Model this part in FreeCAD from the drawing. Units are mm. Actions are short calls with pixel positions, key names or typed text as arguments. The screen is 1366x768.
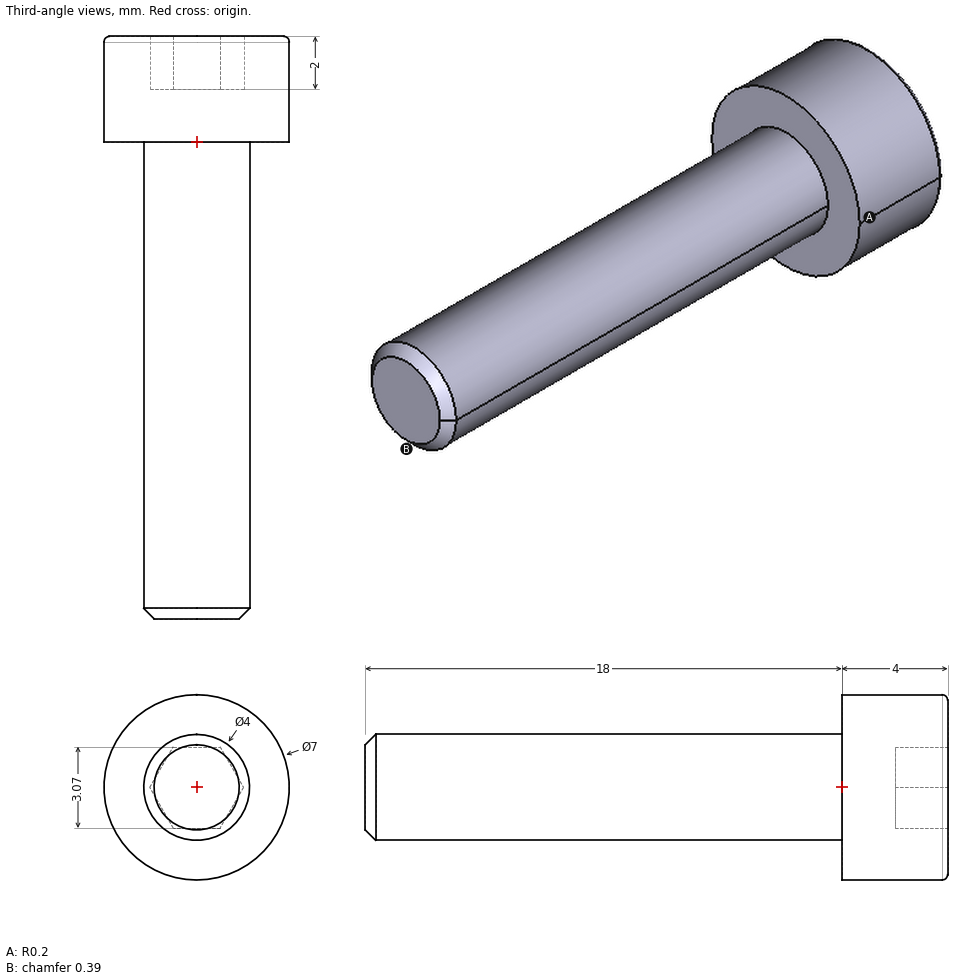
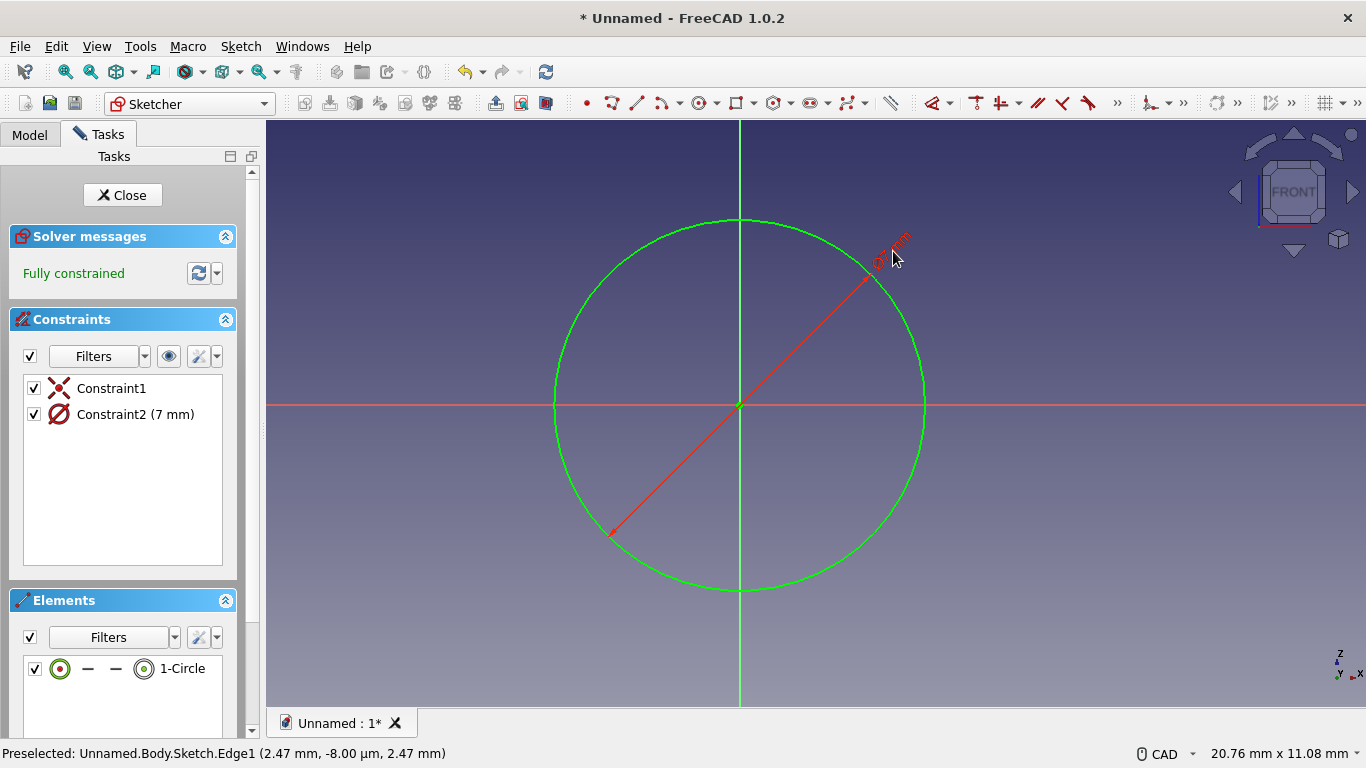
click(123, 195)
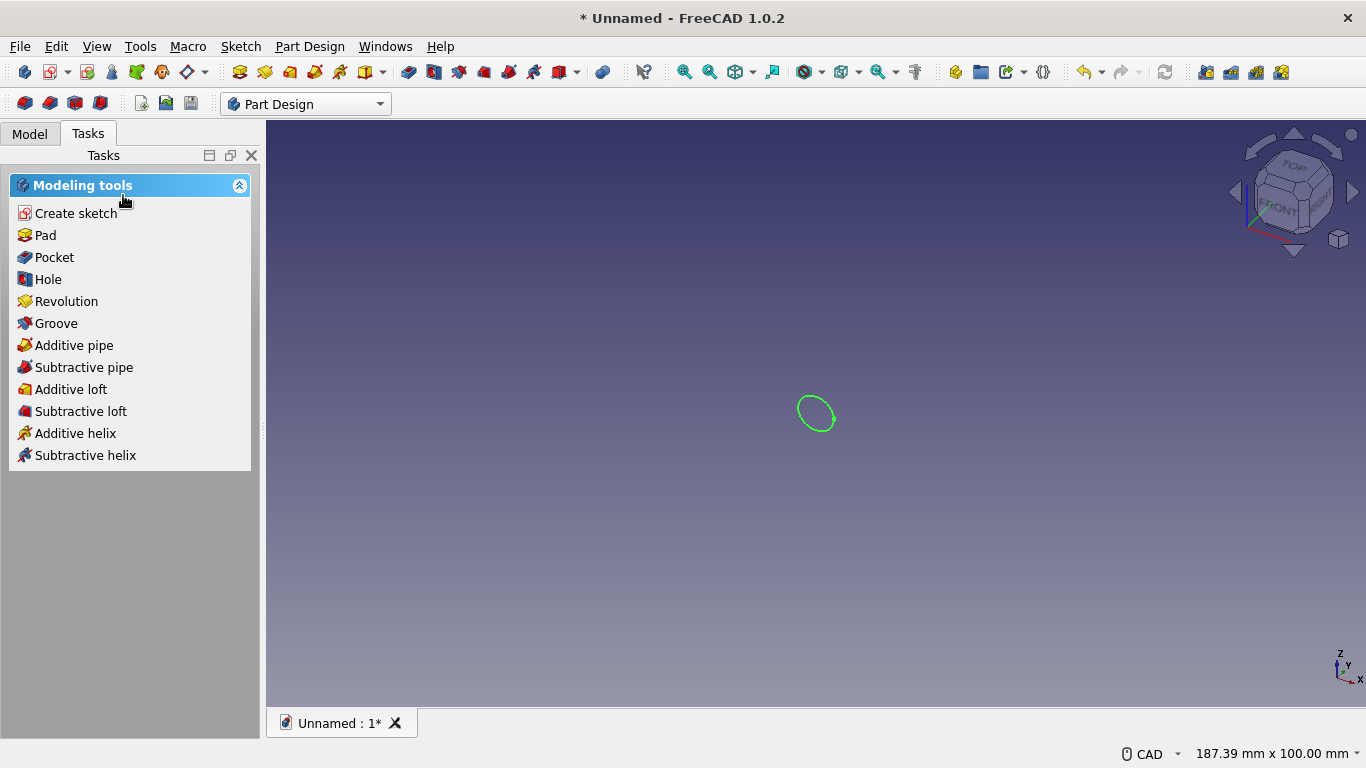
click(240, 72)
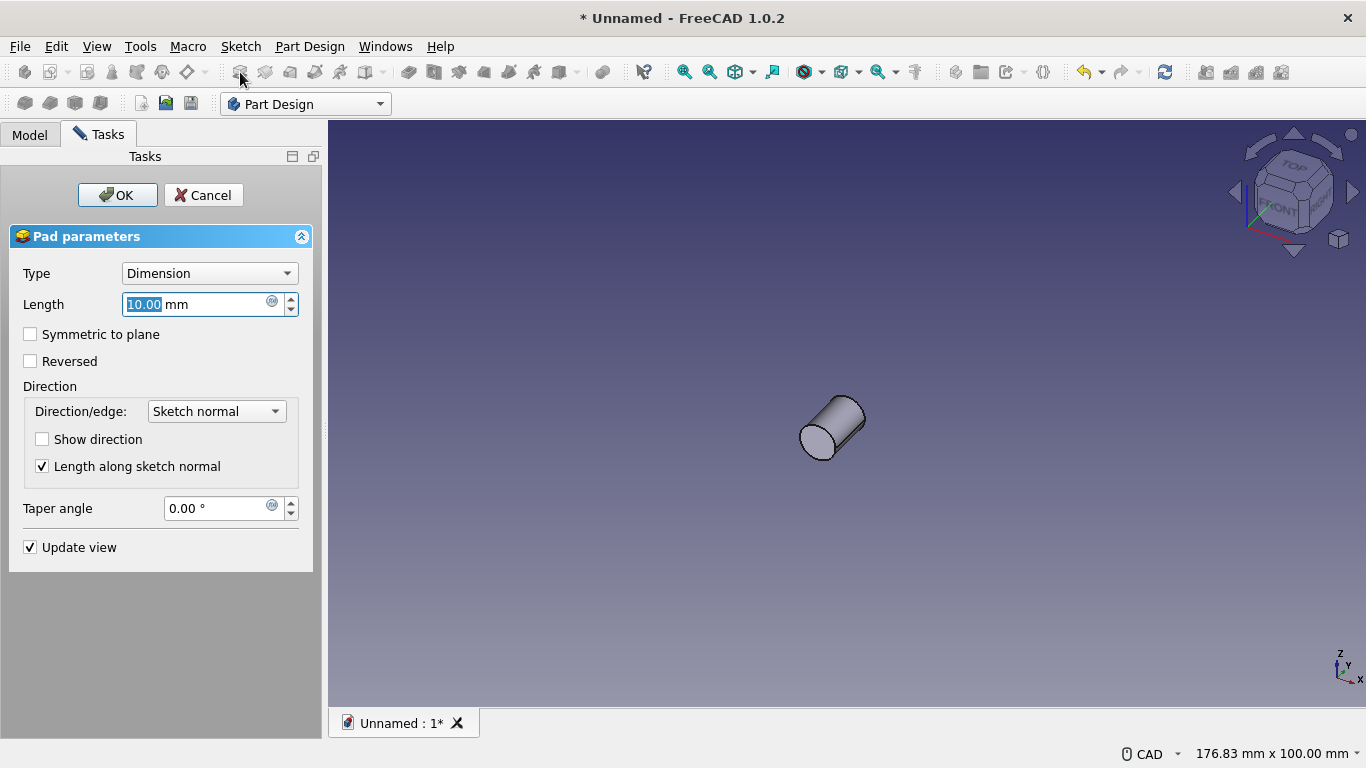
text(4)
key(Tab)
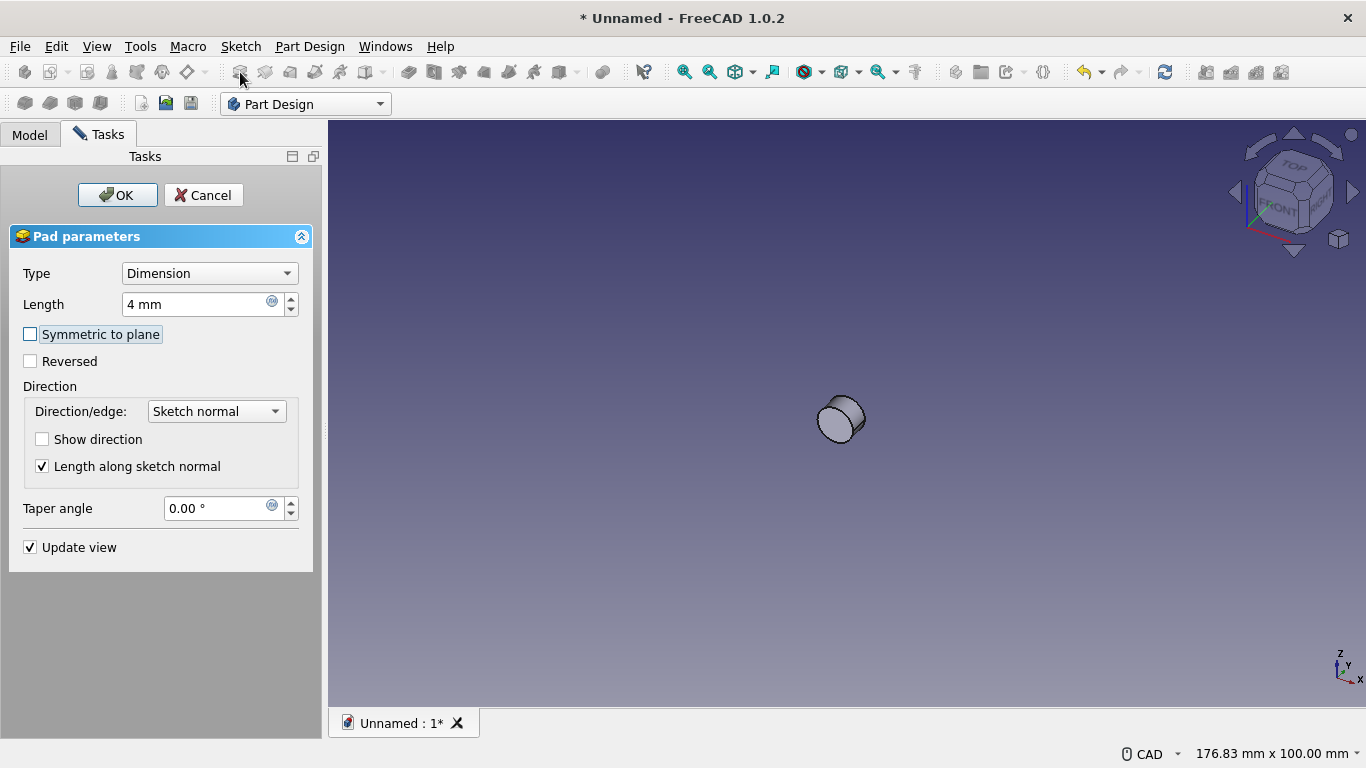
click(31, 361)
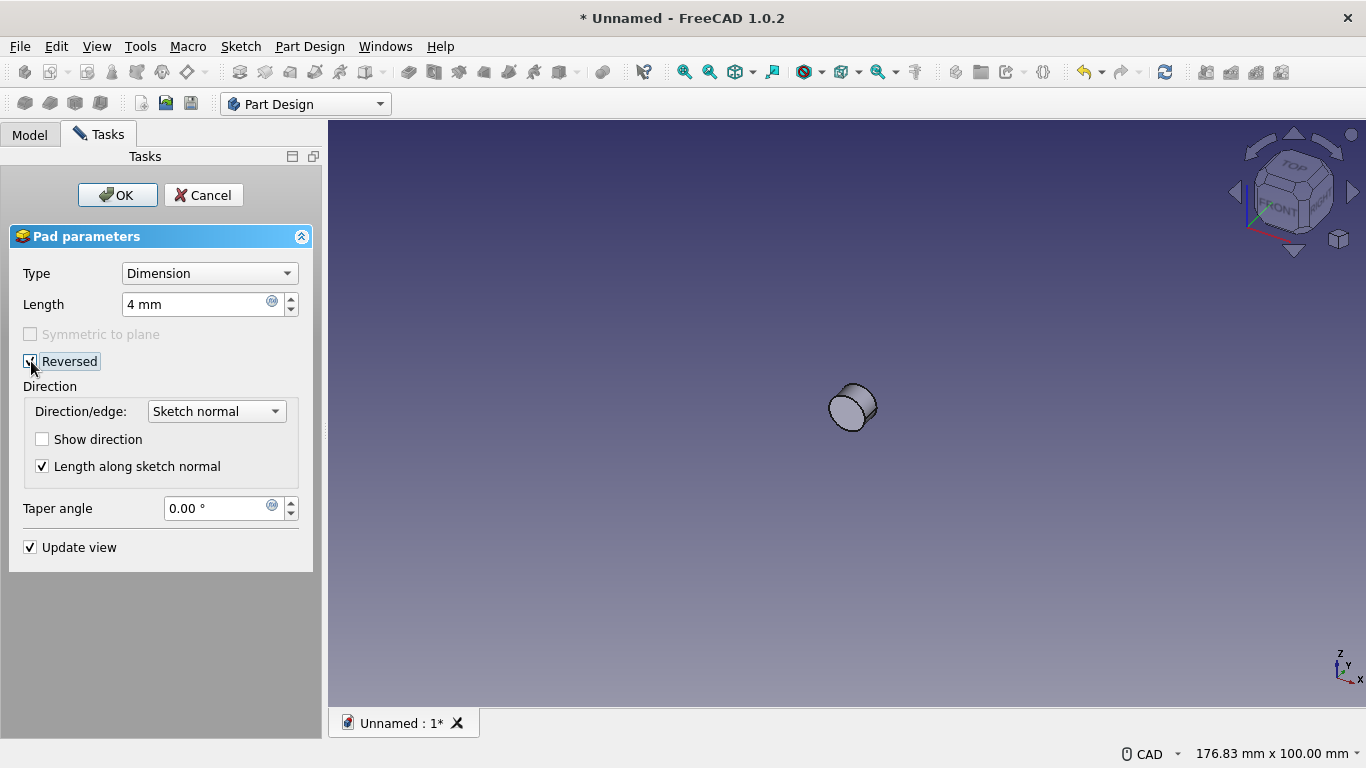
click(118, 195)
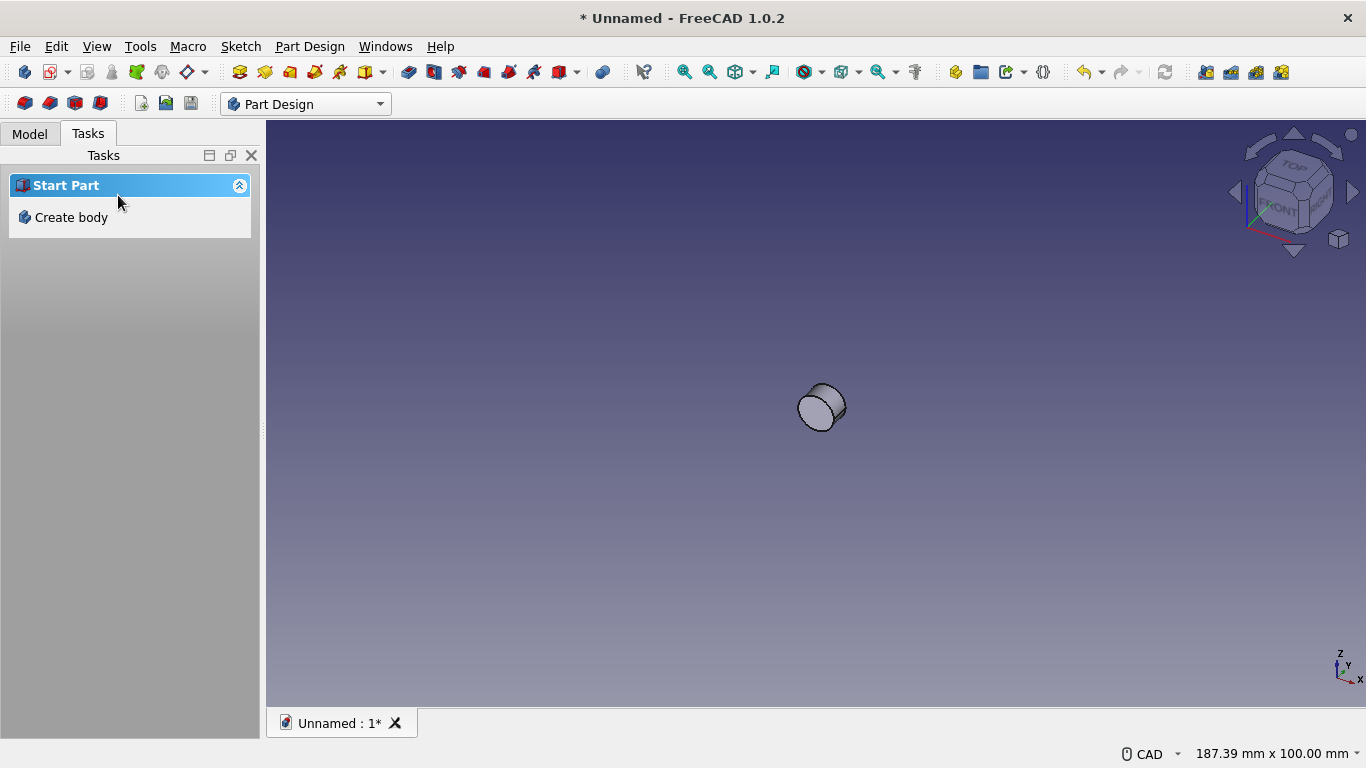
click(685, 72)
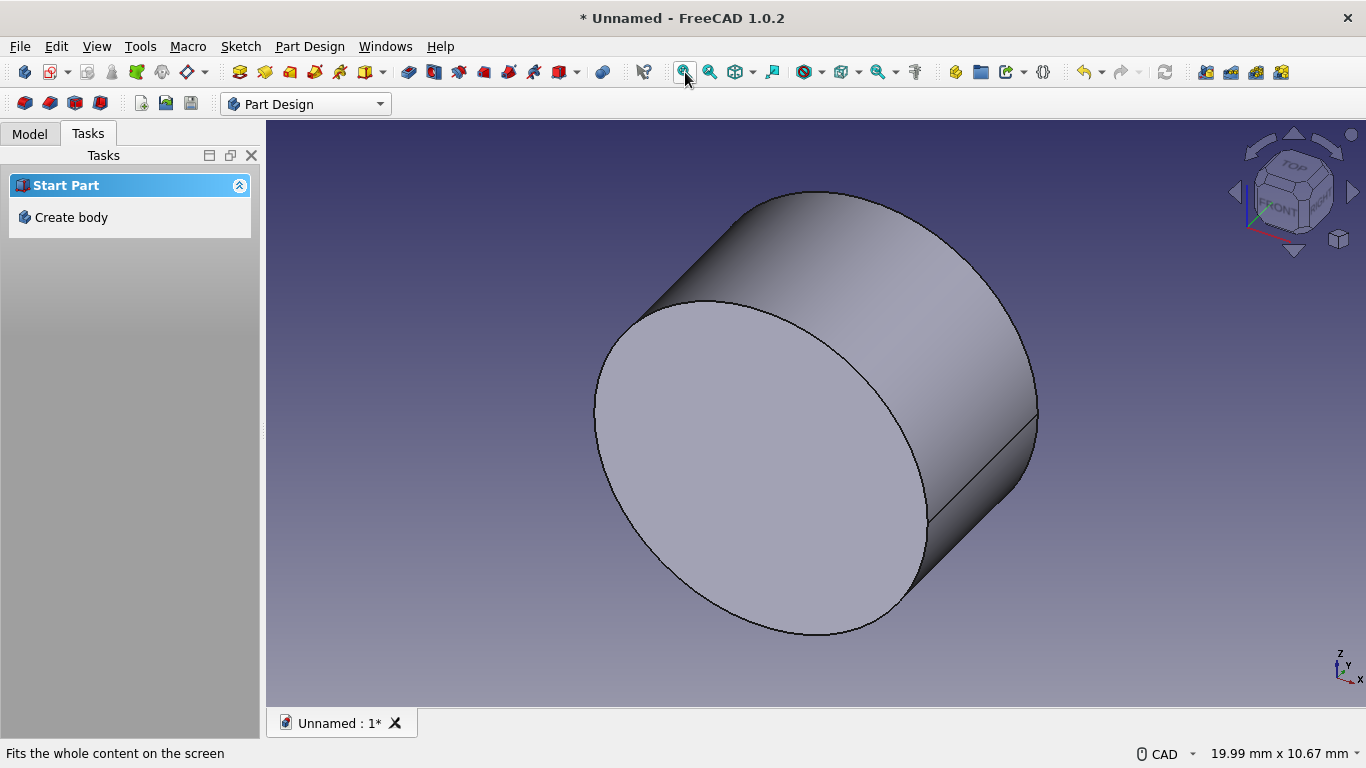
key(4)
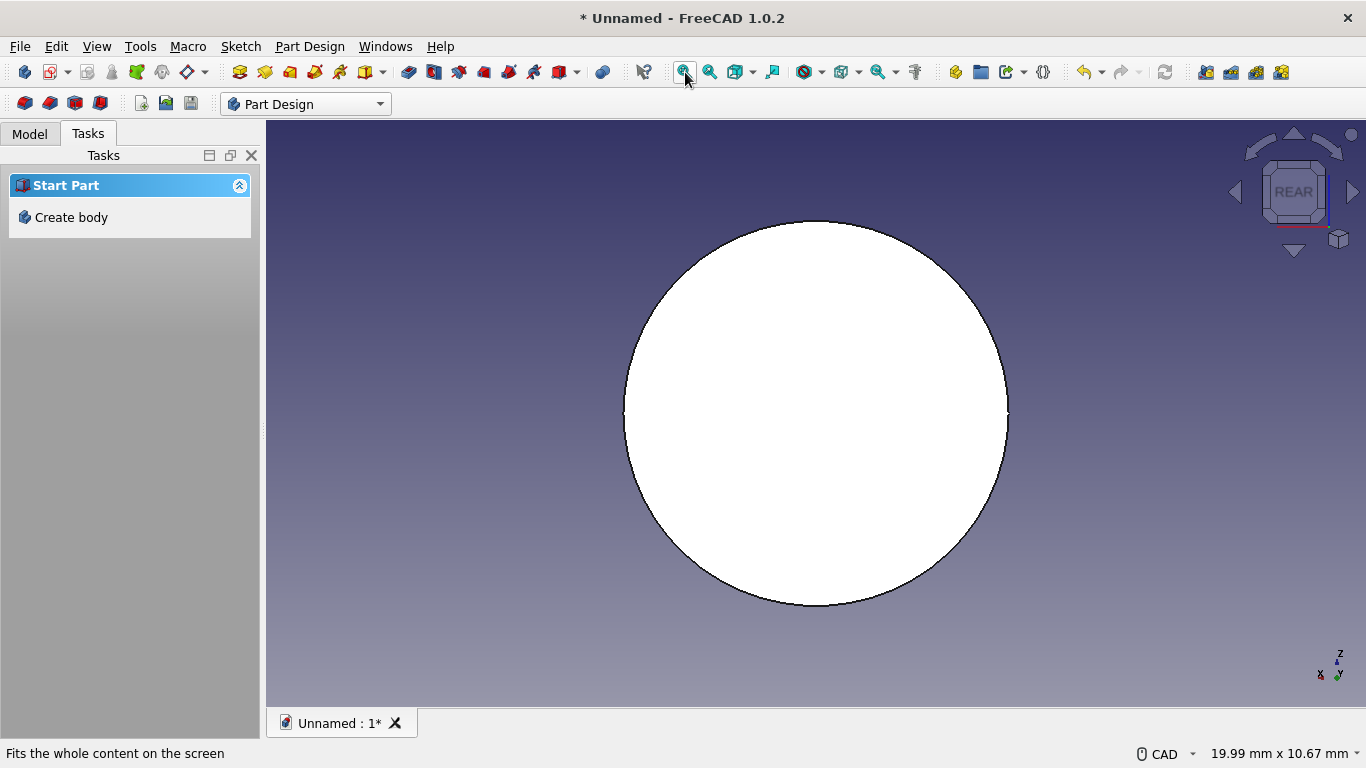
click(816, 413)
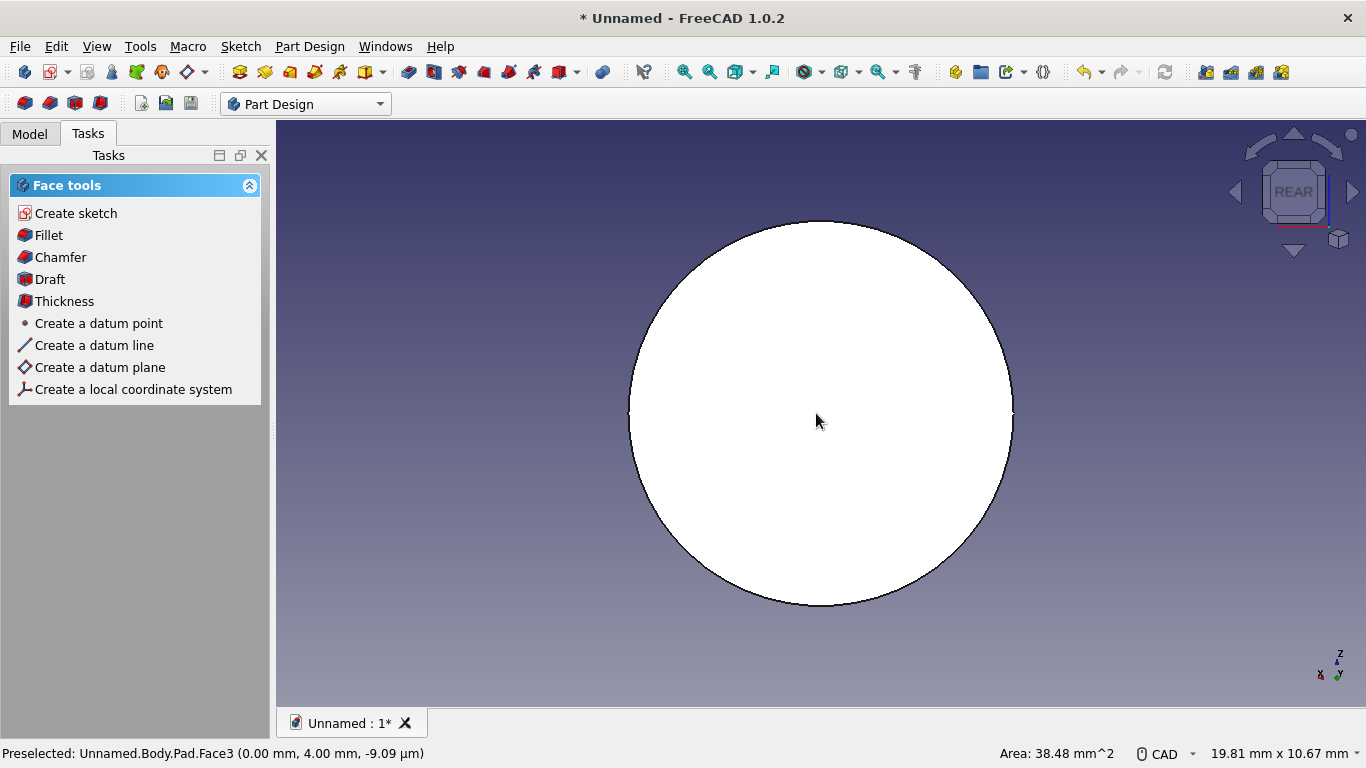
click(50, 72)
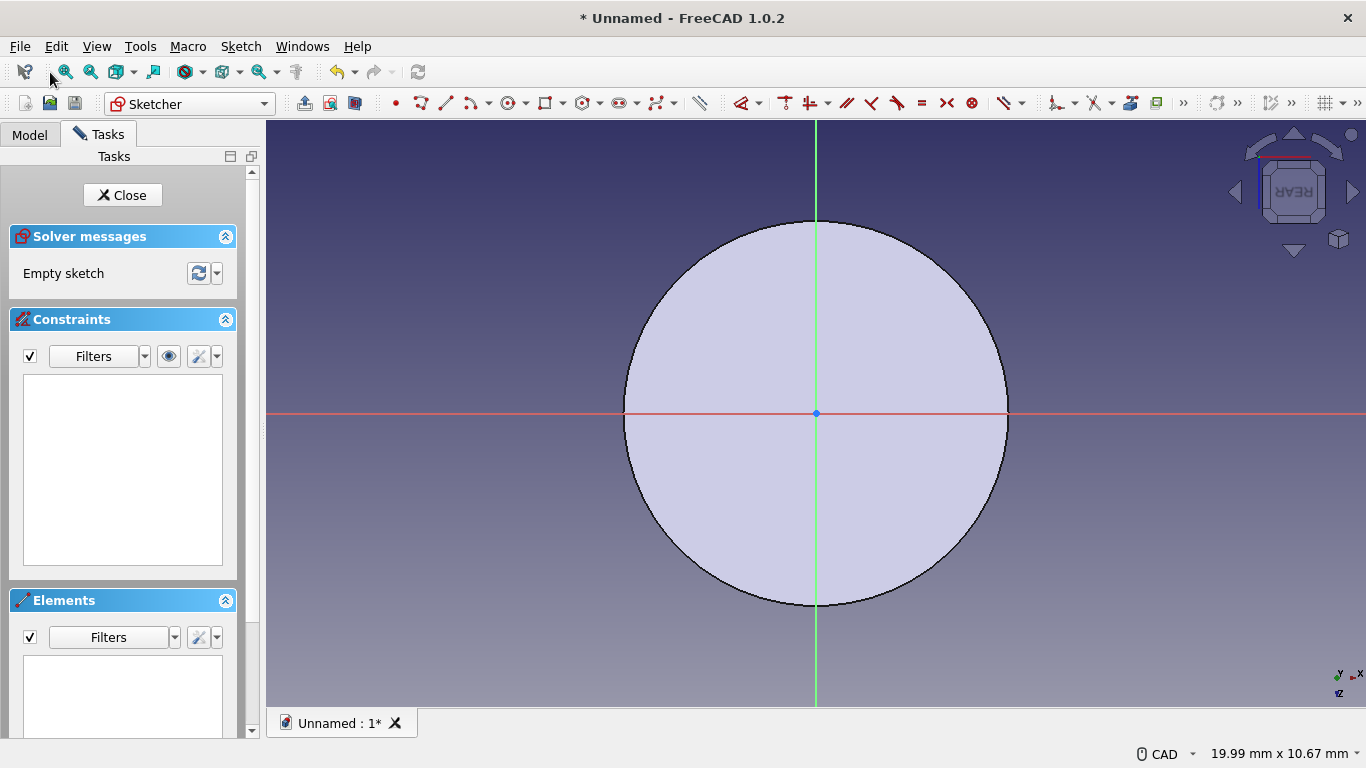
scroll(872, 414, up, 4)